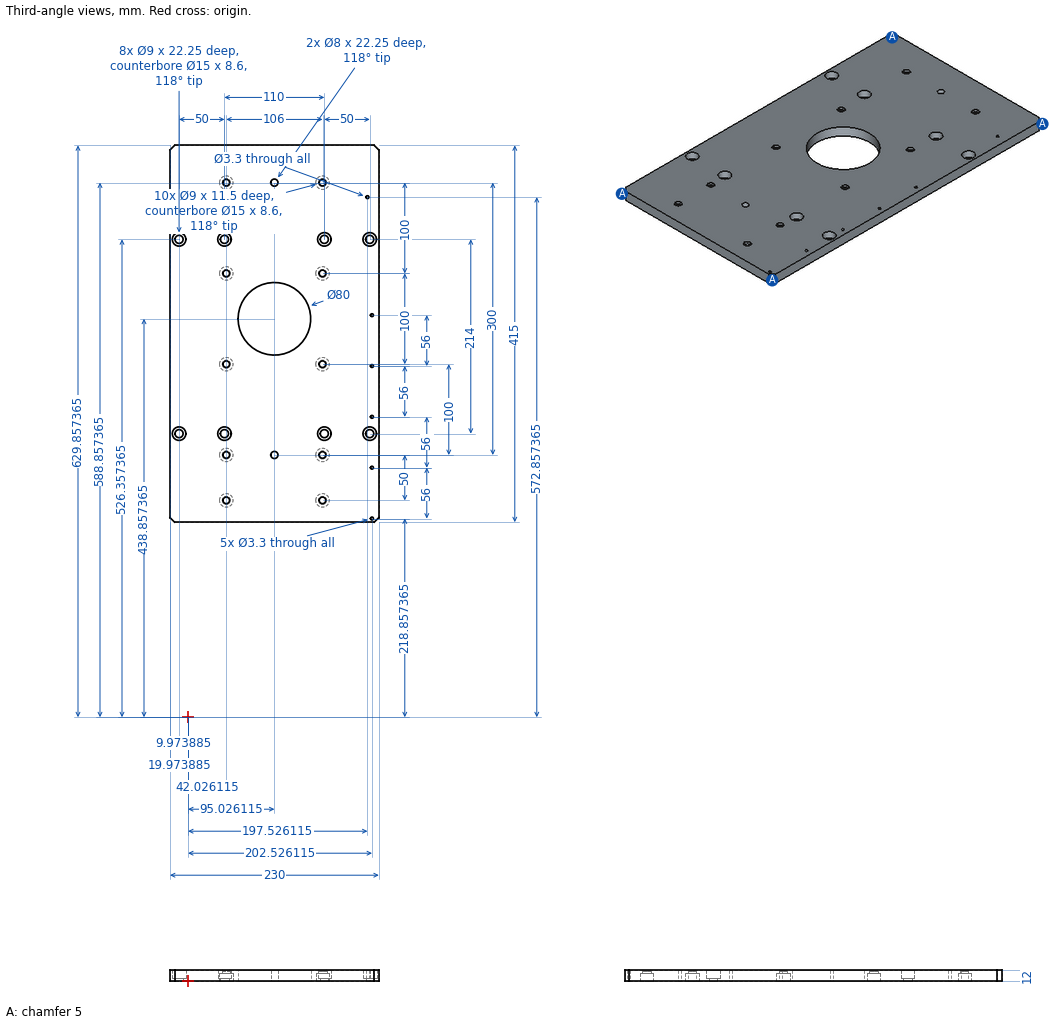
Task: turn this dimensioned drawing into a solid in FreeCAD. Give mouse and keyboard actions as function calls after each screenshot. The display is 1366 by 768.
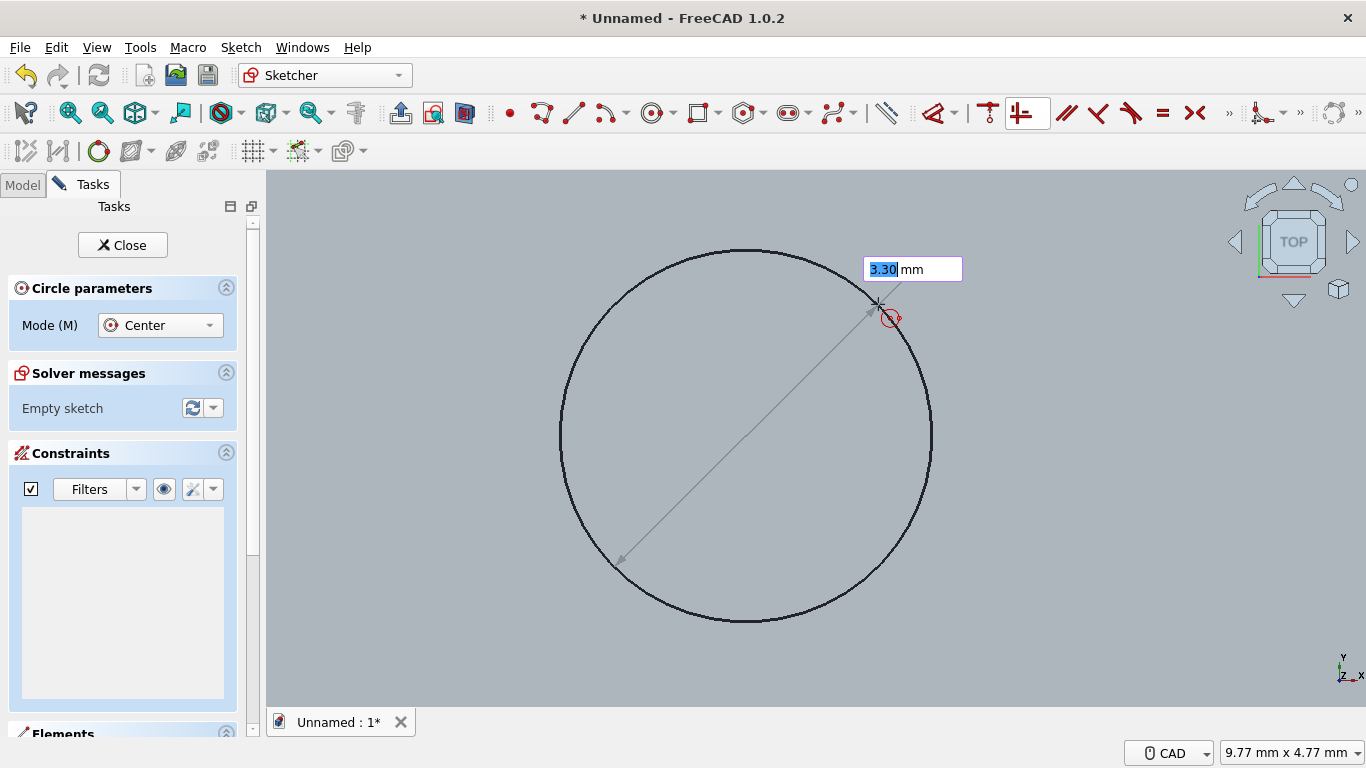
text(3.3)
key(Return)
key(Escape)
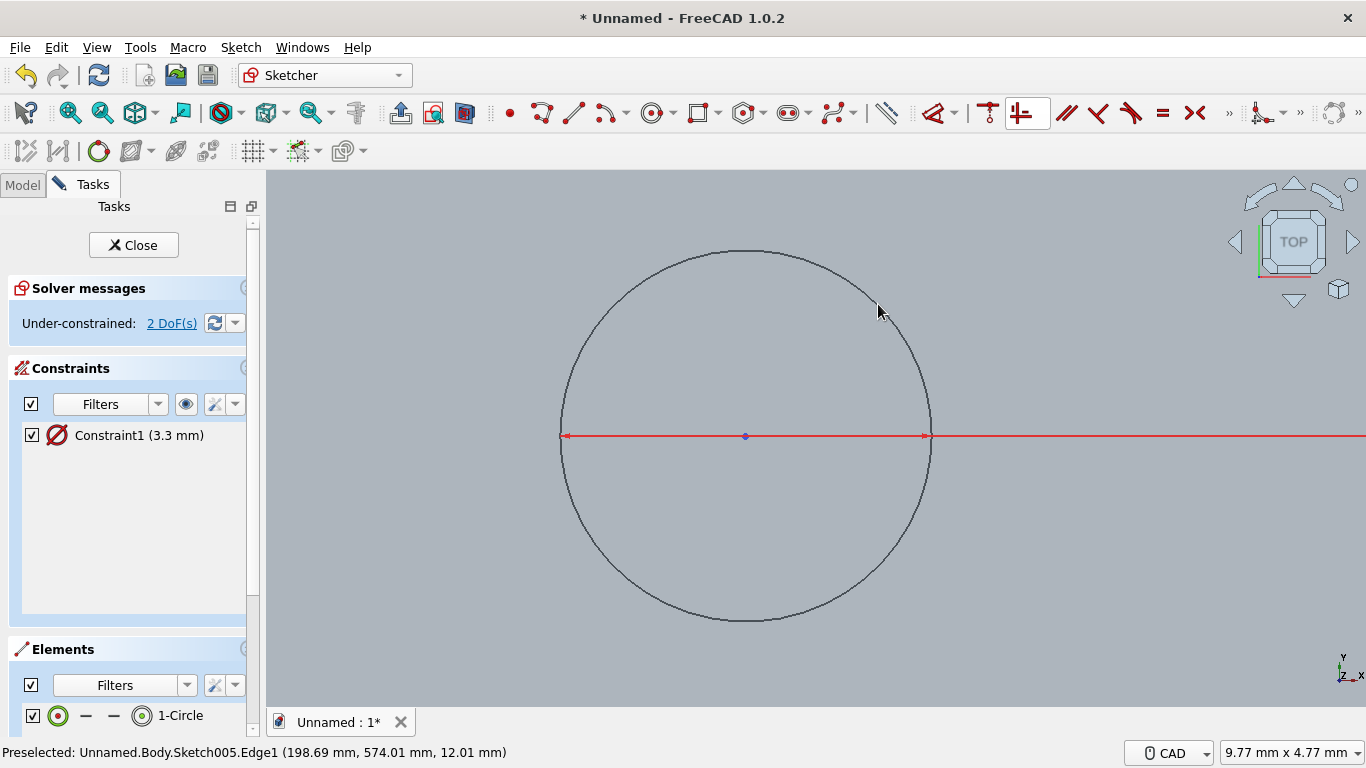
click(934, 114)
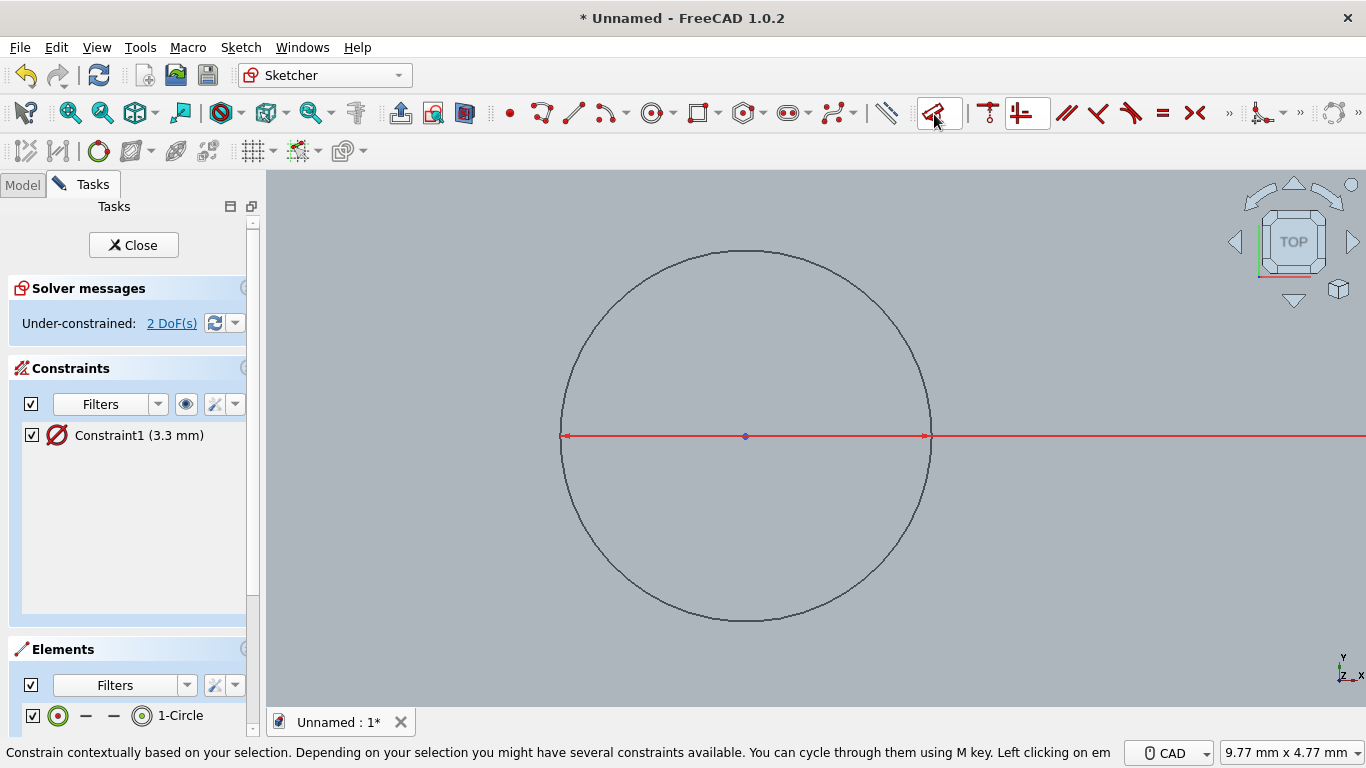
click(746, 436)
click(520, 402)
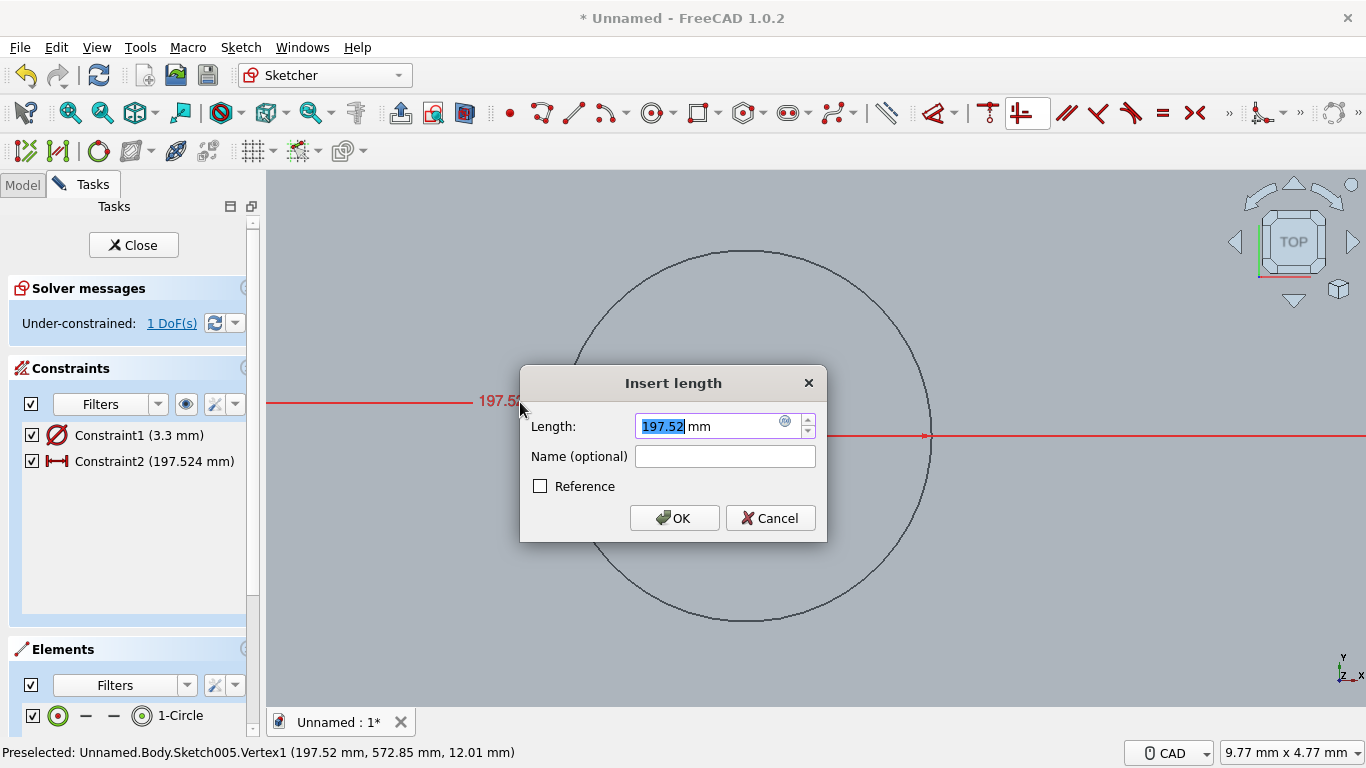
text(197.526115)
key(Return)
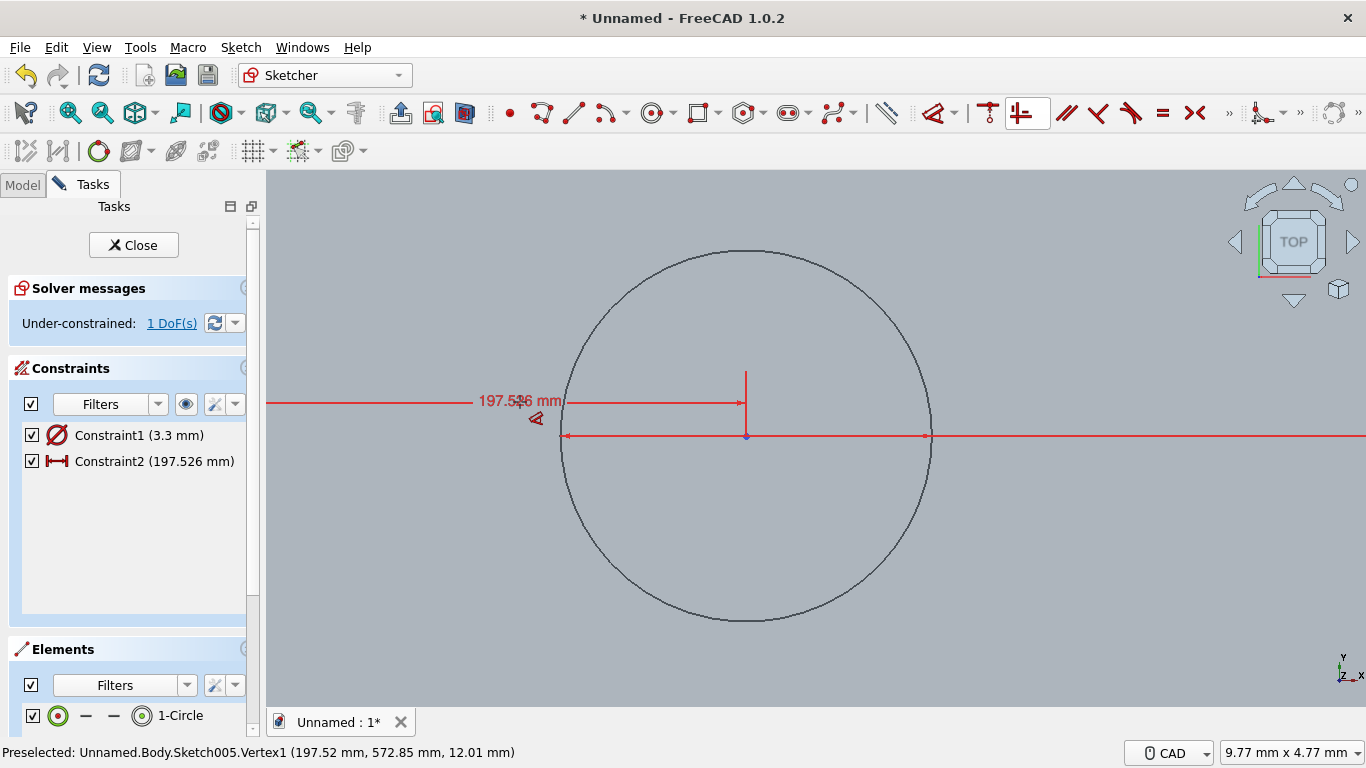
click(746, 436)
click(780, 557)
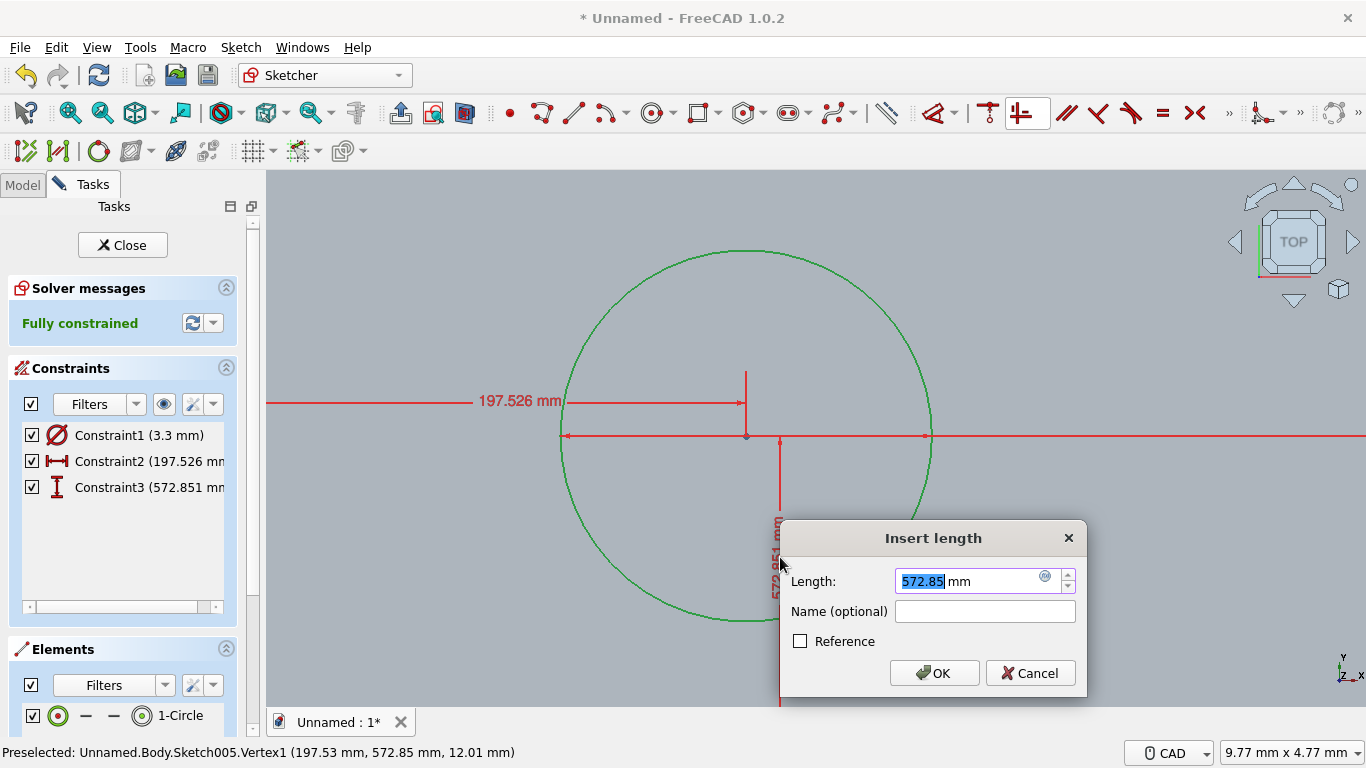
text(572.857365)
key(Return)
key(Escape)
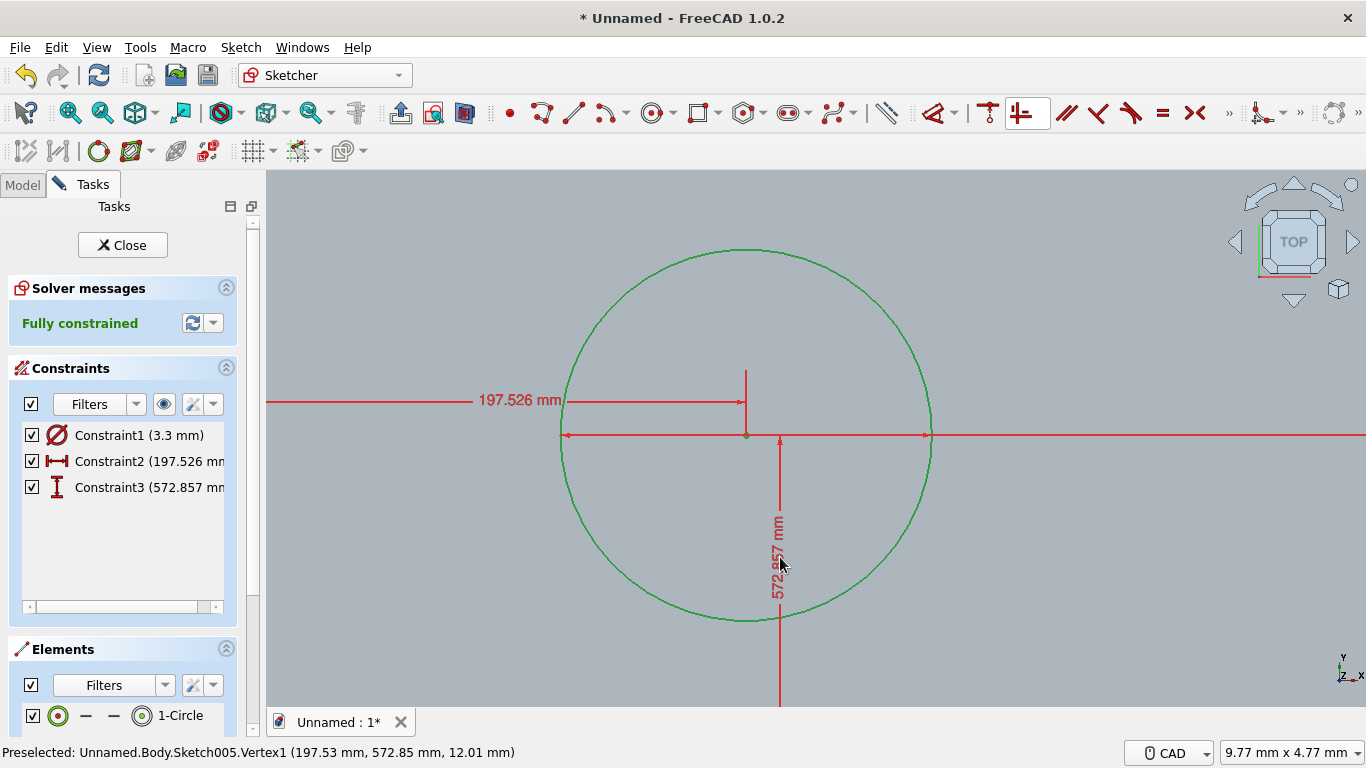
click(123, 245)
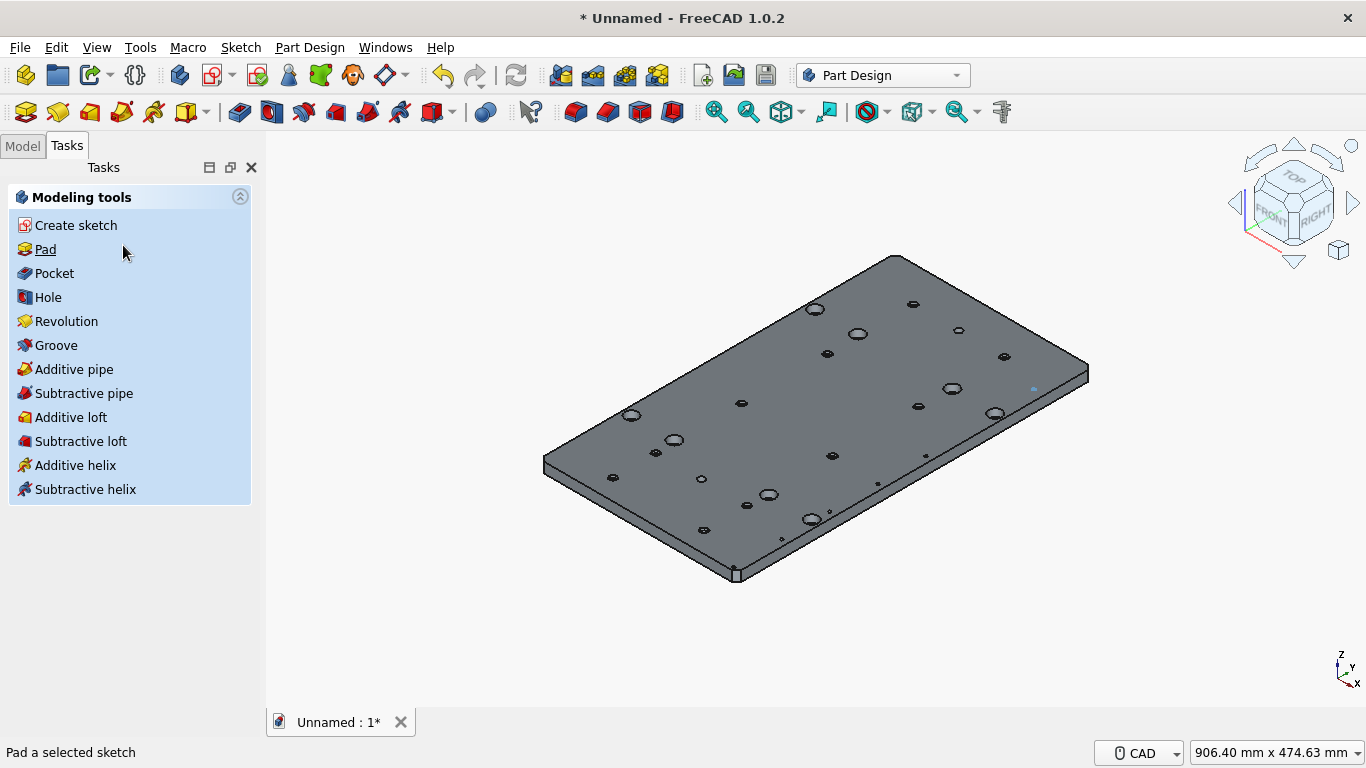
click(272, 112)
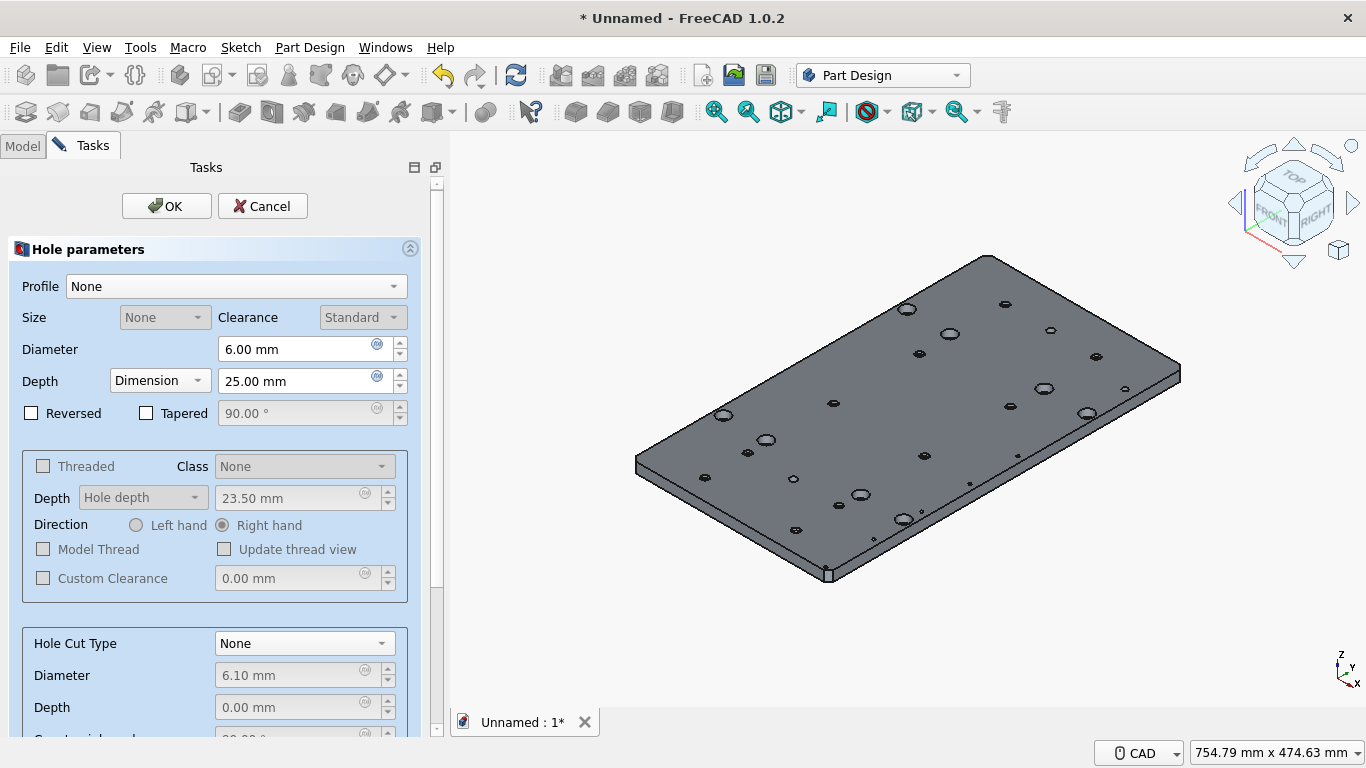
triple_click(305, 349)